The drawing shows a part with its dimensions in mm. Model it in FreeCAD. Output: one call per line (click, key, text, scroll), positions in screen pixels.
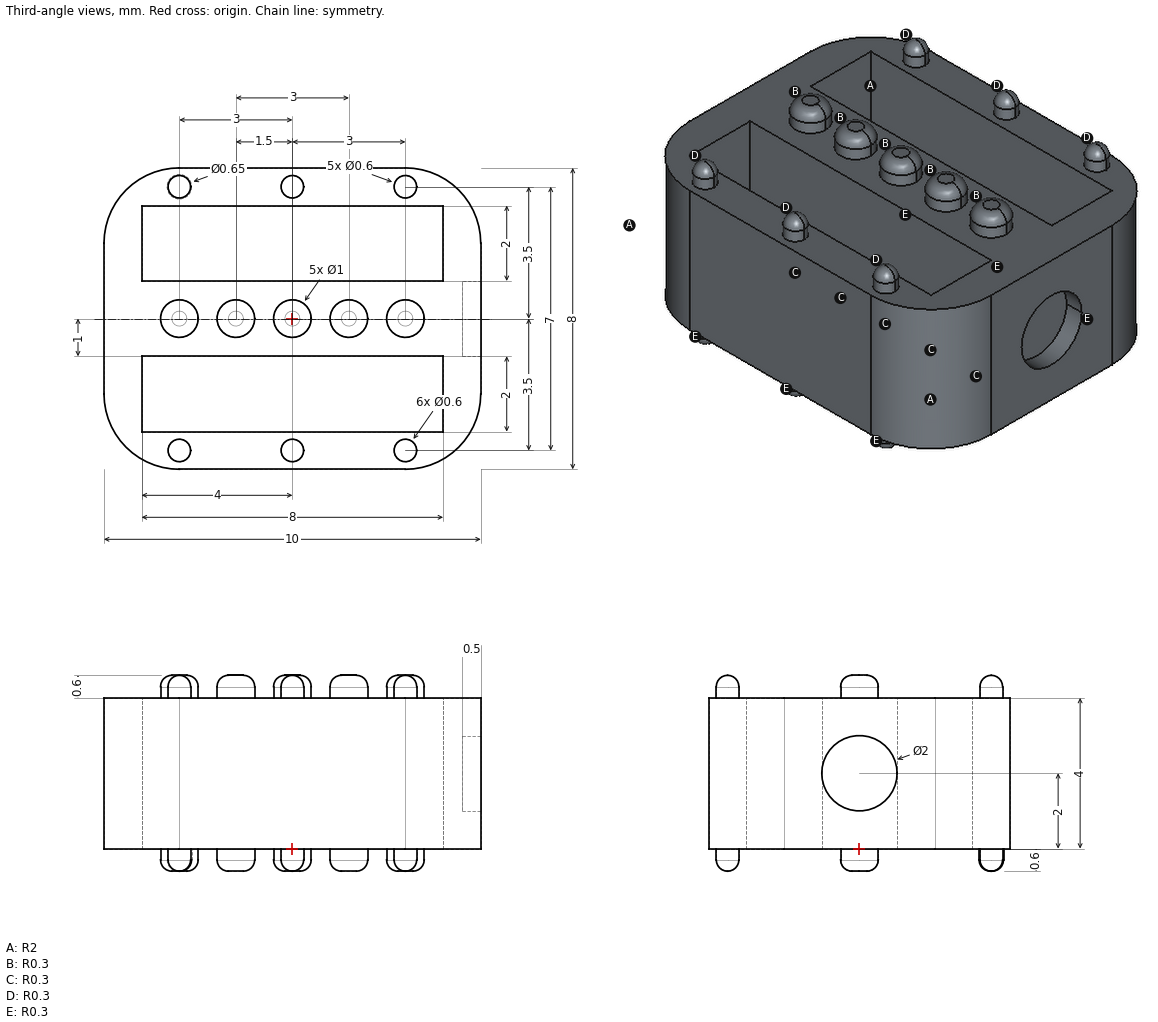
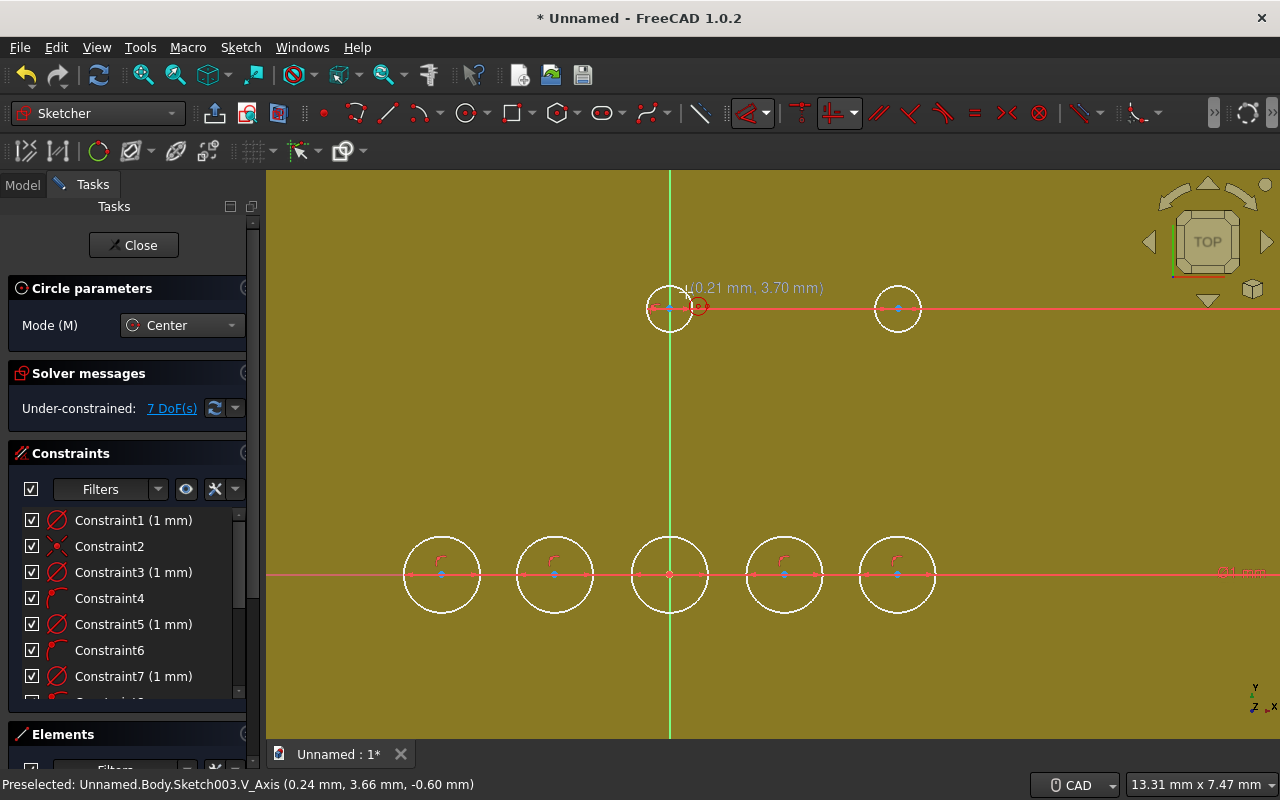
click(441, 308)
move(459, 291)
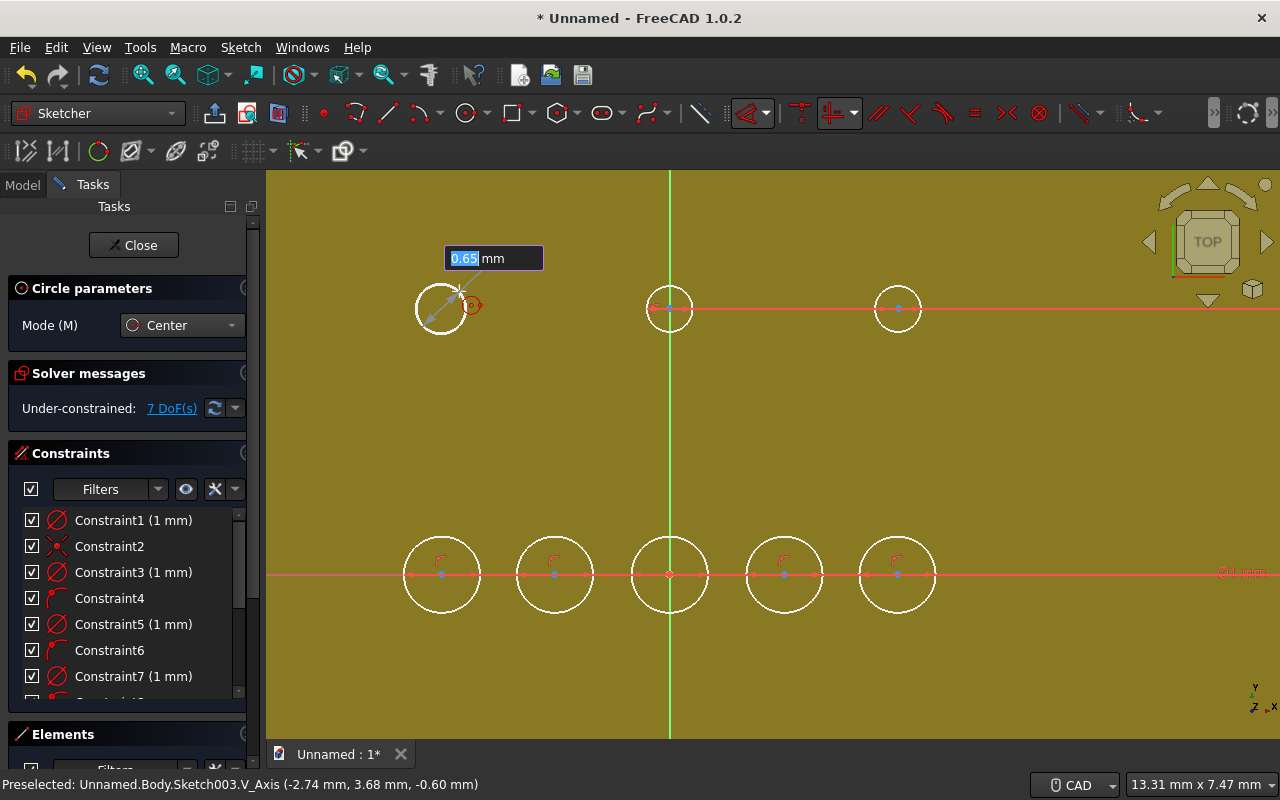
text(0.65)
key(Return)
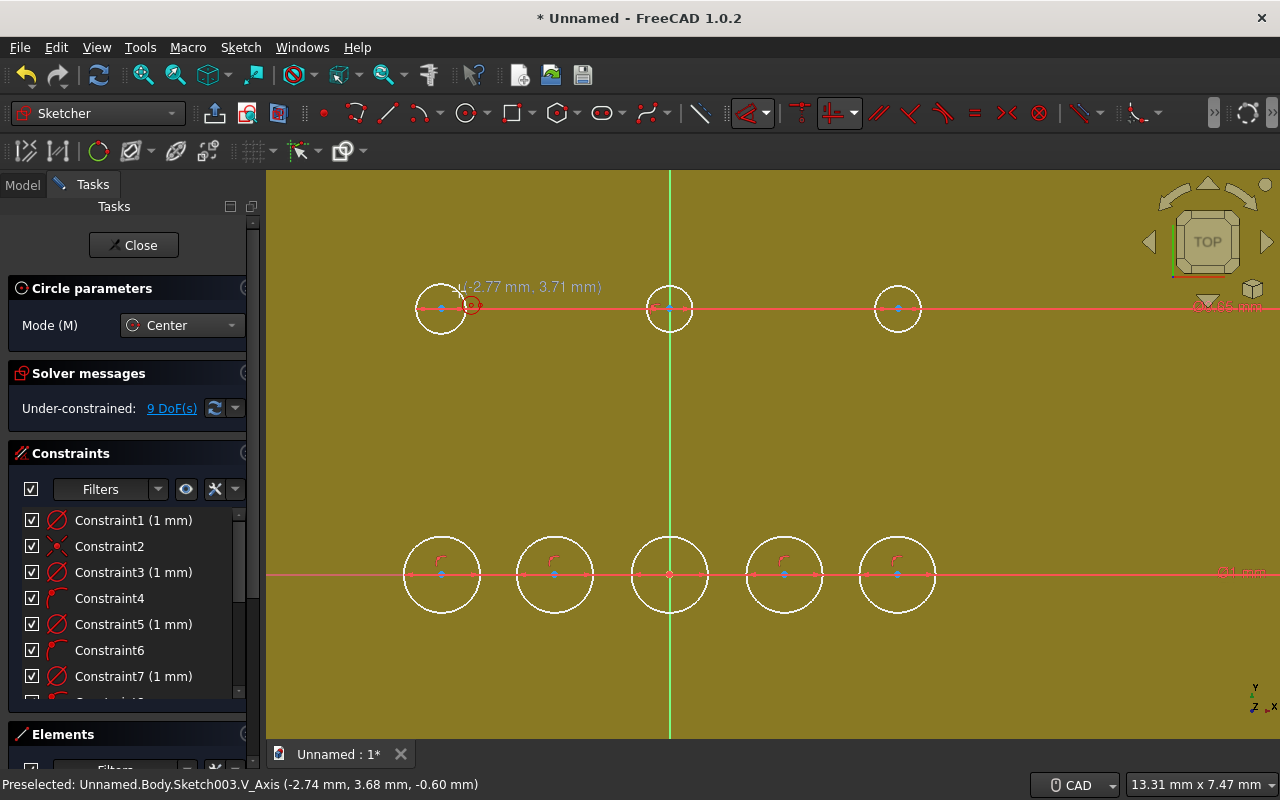
scroll(775, 212, down, 2)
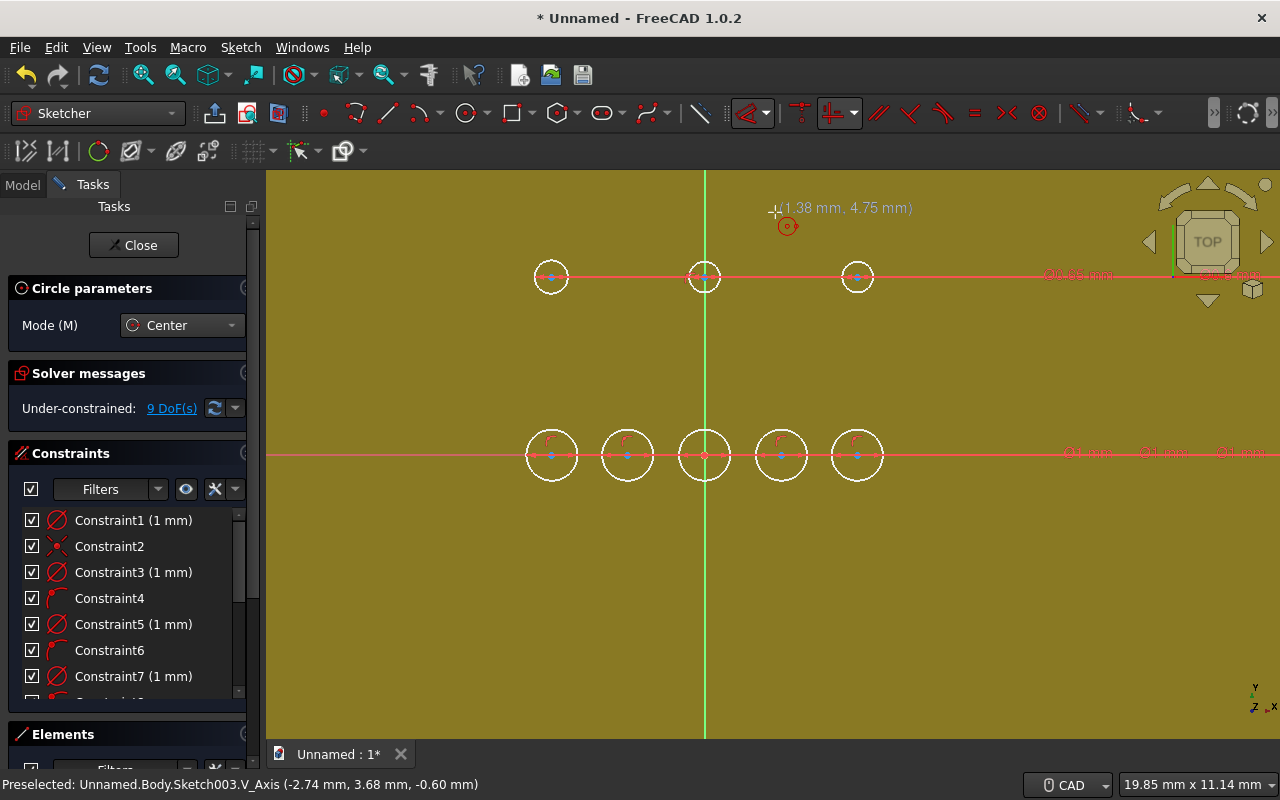
scroll(858, 634, up, 2)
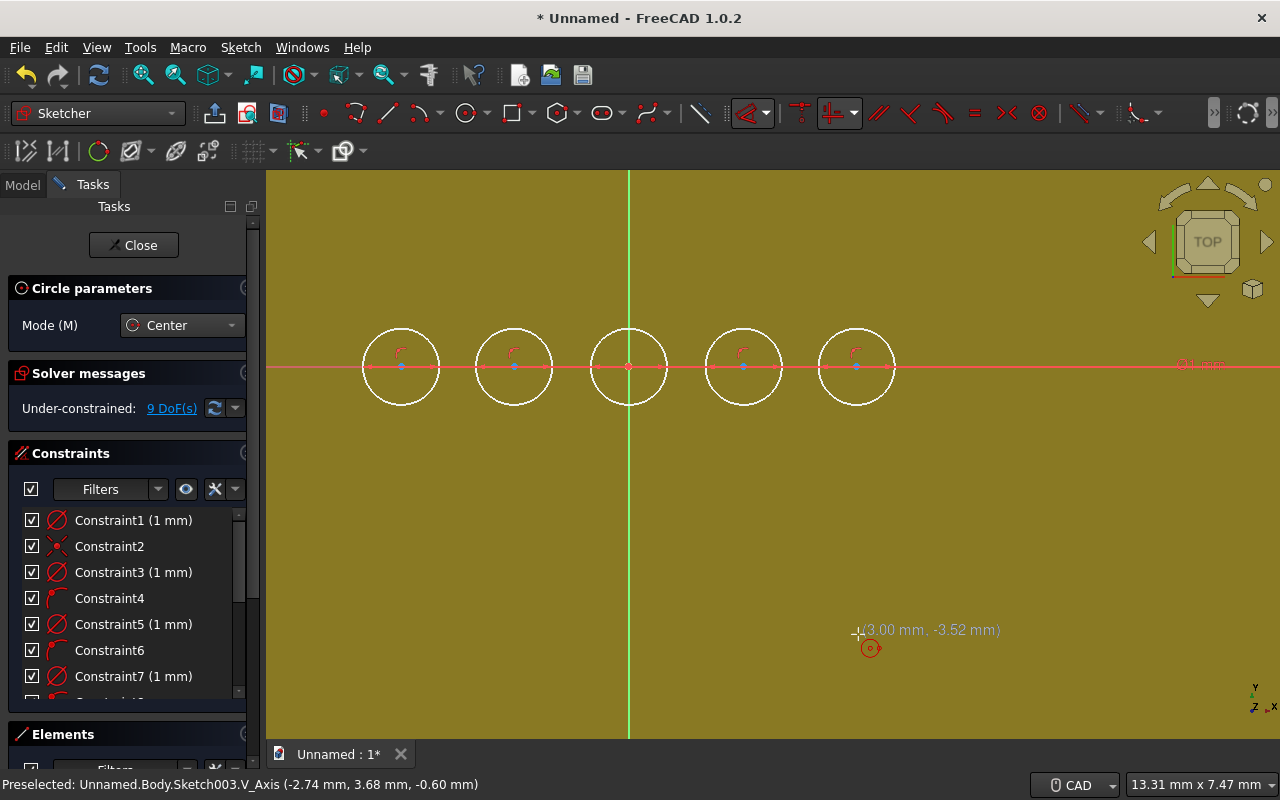
click(857, 634)
move(874, 617)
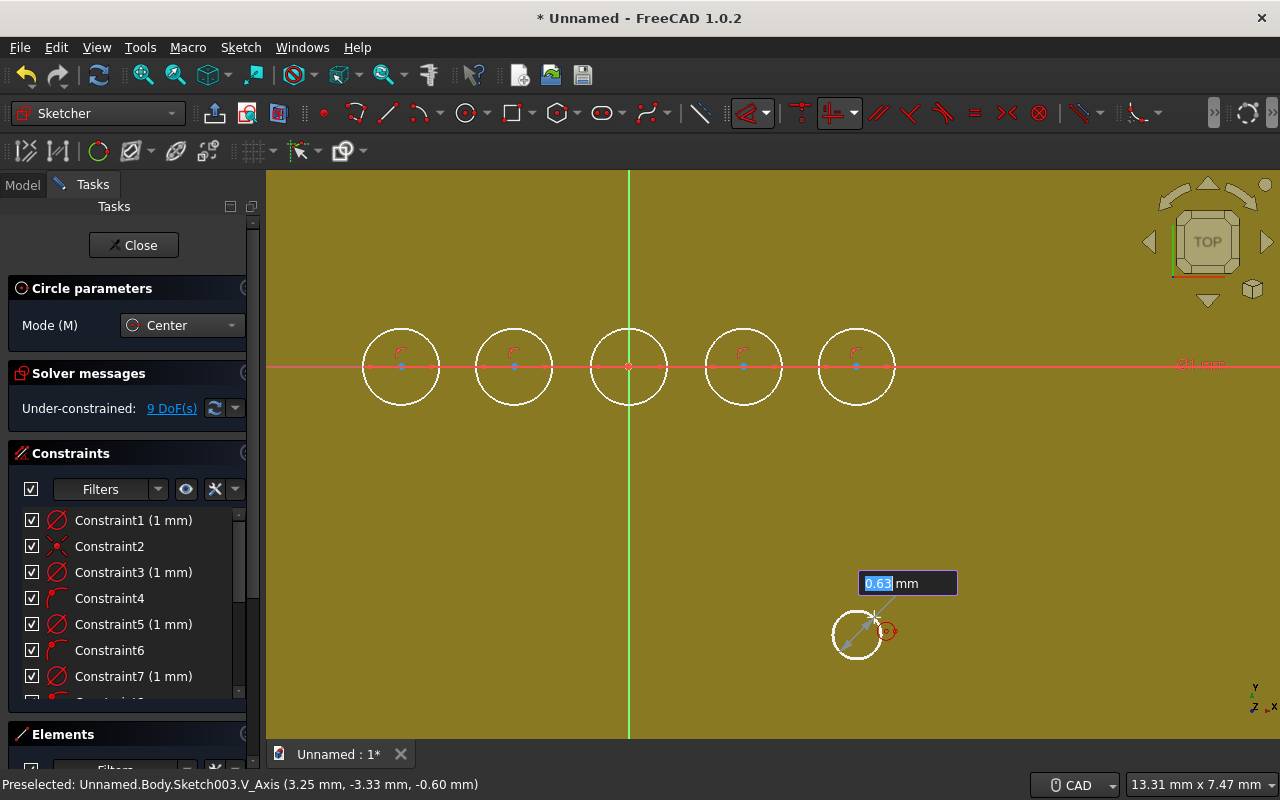
text(0.6)
key(Return)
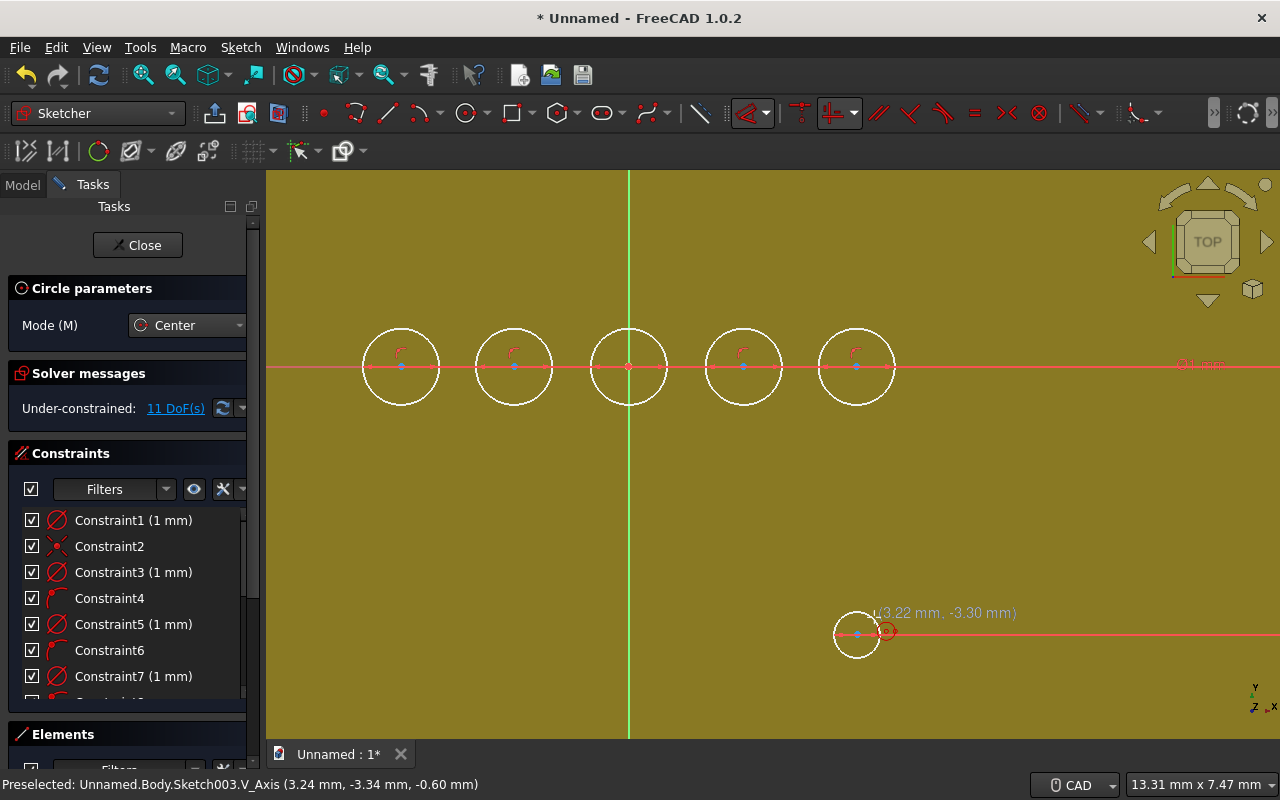
click(629, 634)
move(645, 617)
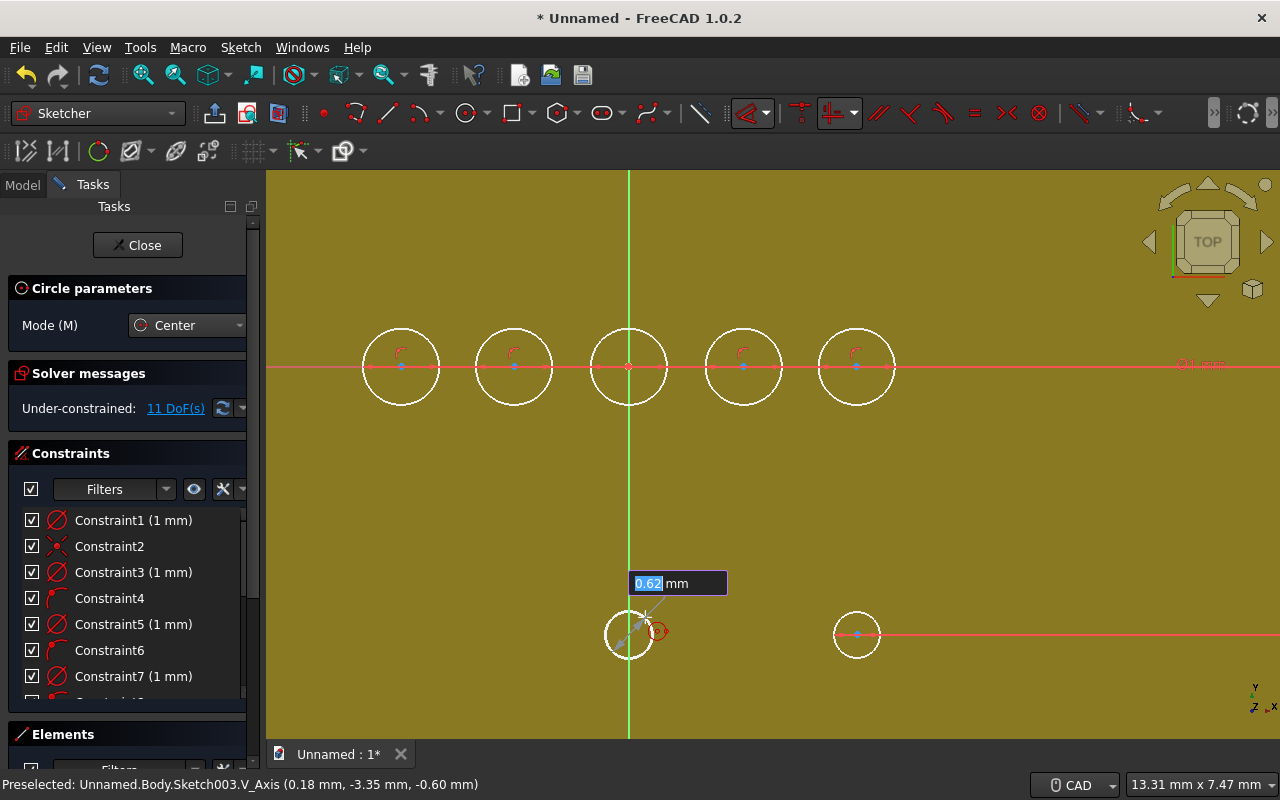
text(0.6)
key(Return)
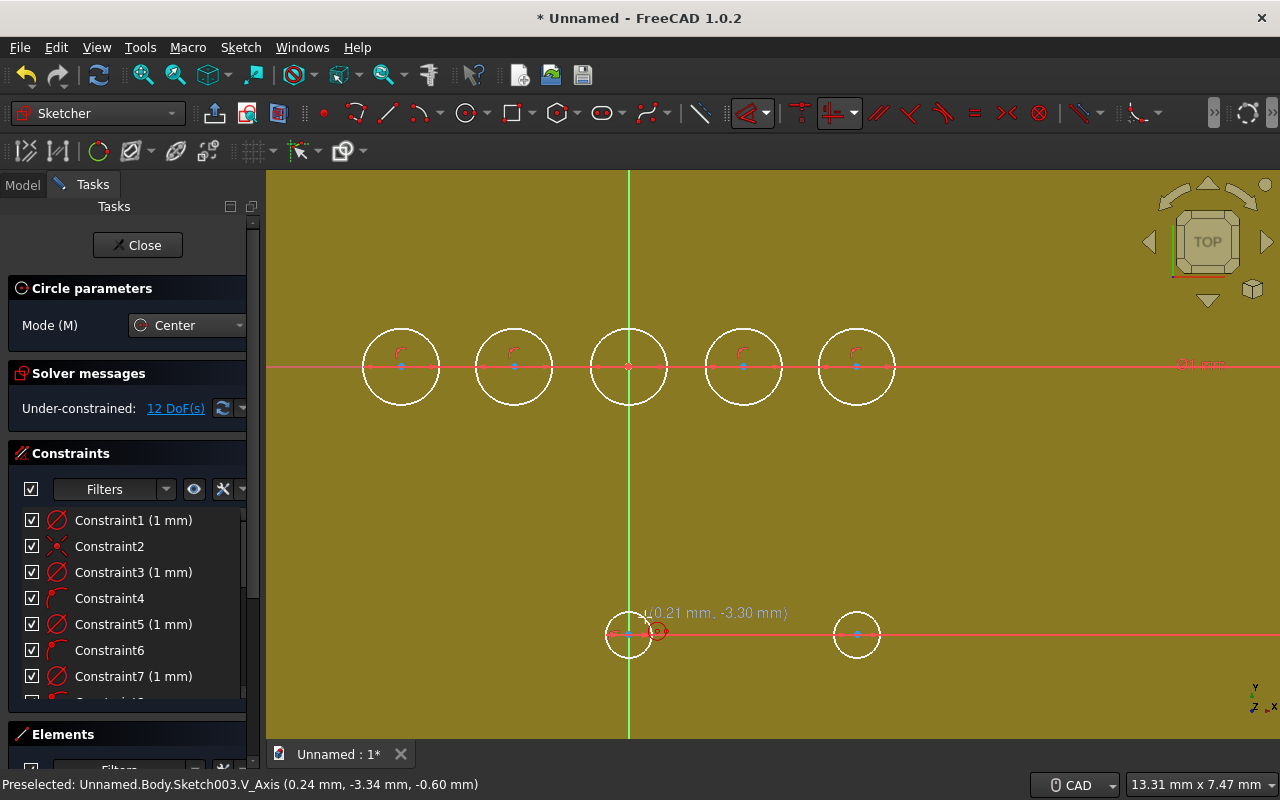
click(400, 634)
move(416, 617)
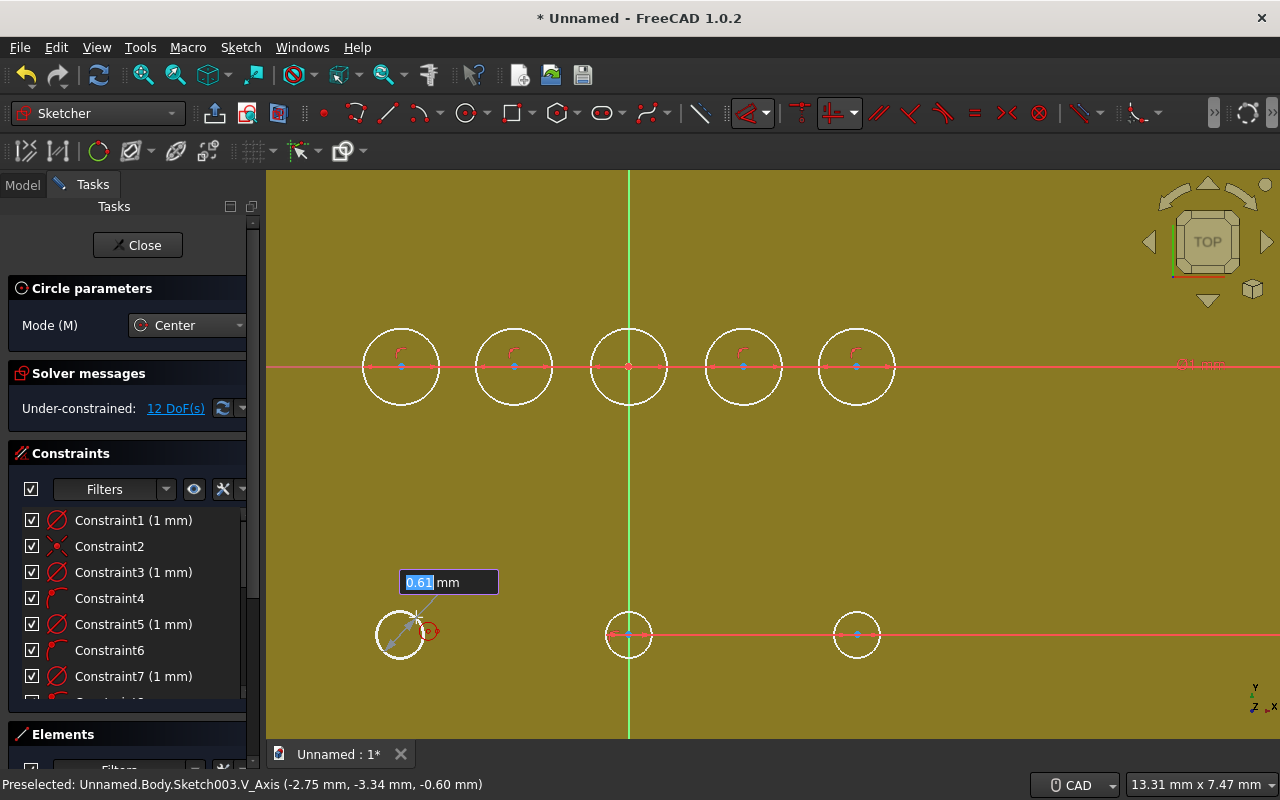
text(0.6)
key(Return)
key(Escape)